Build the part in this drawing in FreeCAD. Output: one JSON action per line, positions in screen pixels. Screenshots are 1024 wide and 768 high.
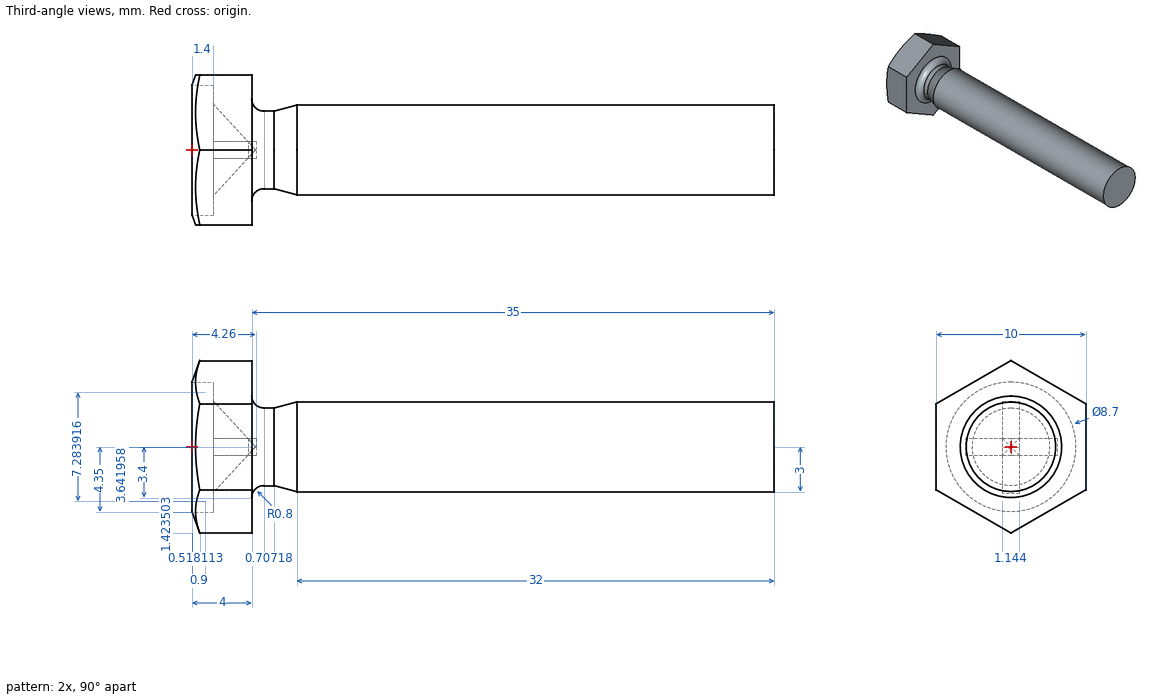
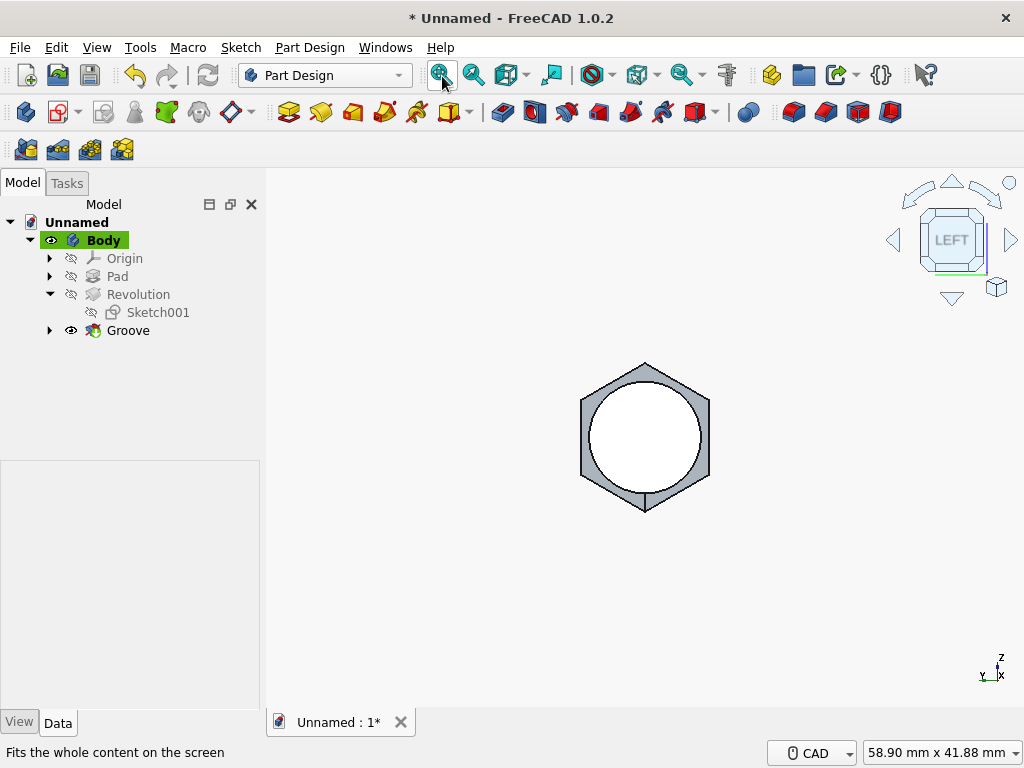
{"action": "key", "text": "v f"}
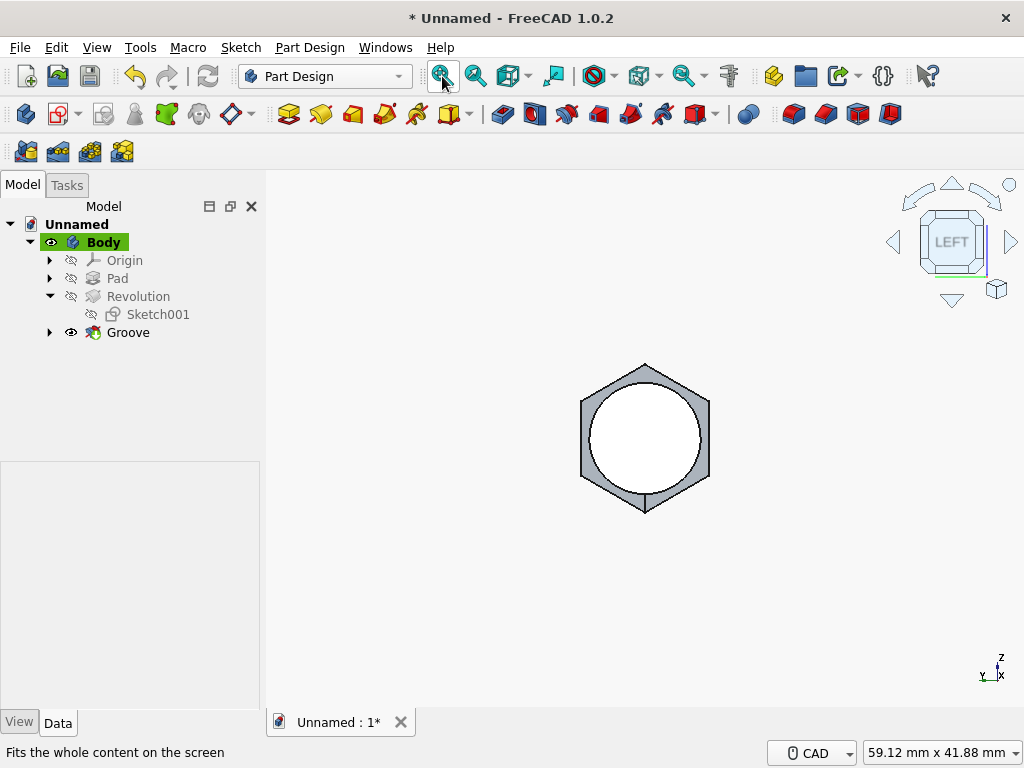
{"action": "left_click", "coordinate": [645, 437]}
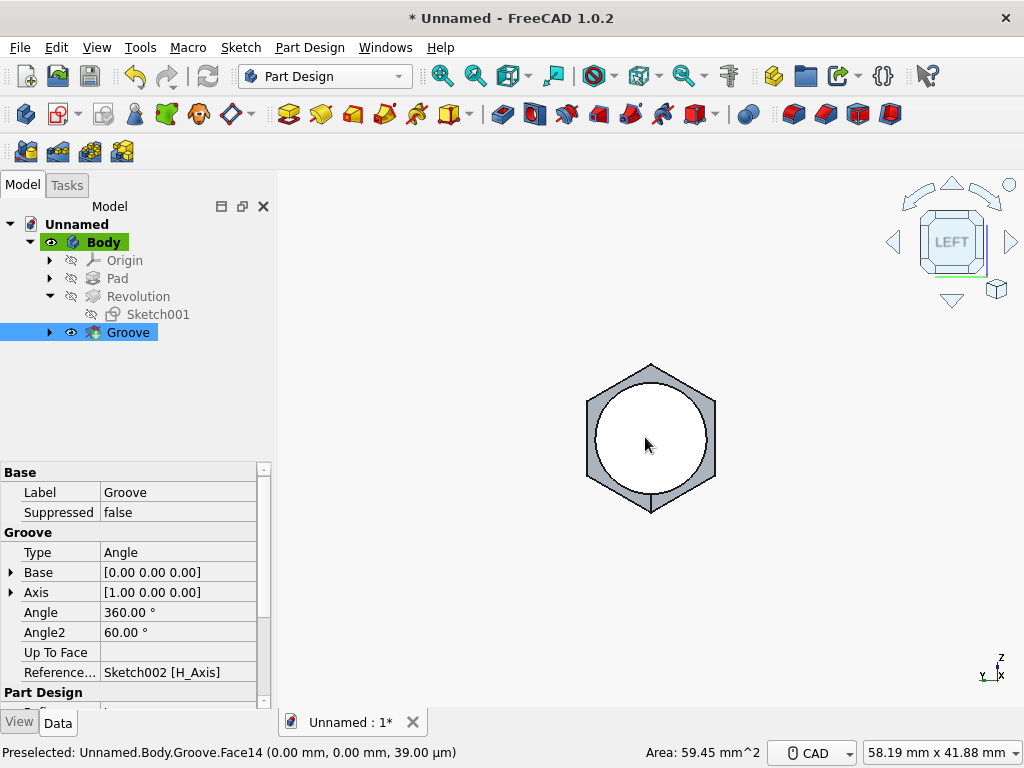
{"action": "left_click", "coordinate": [58, 114]}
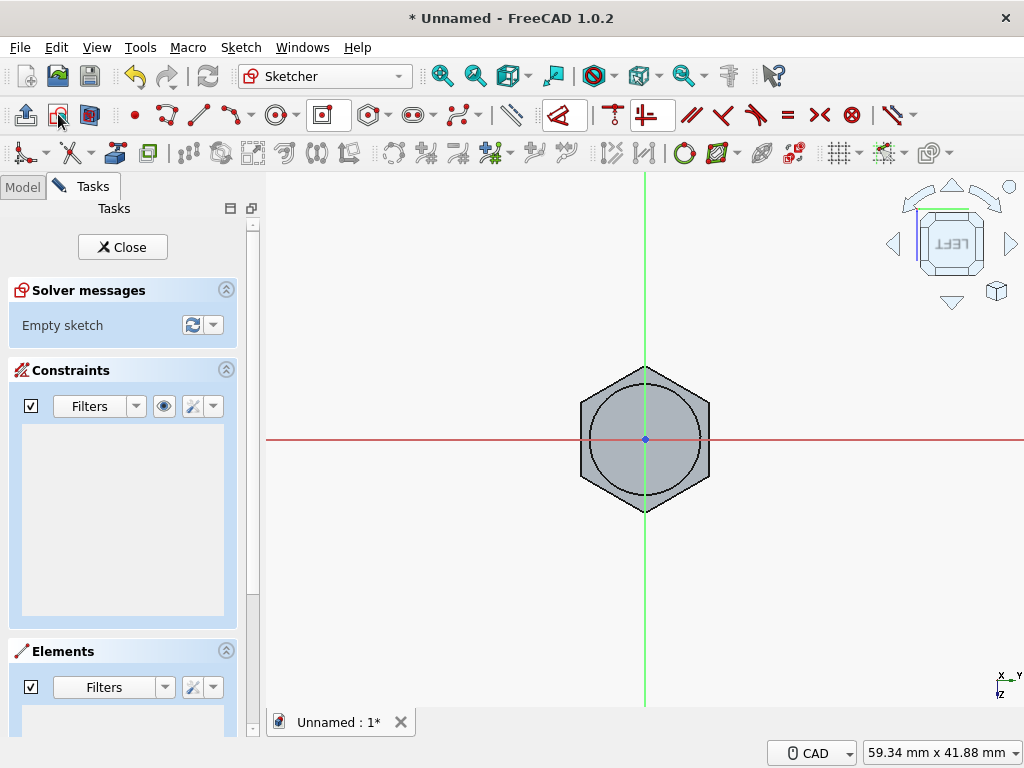
{"action": "scroll", "coordinate": [675, 440], "scroll_direction": "up", "scroll_amount": 6}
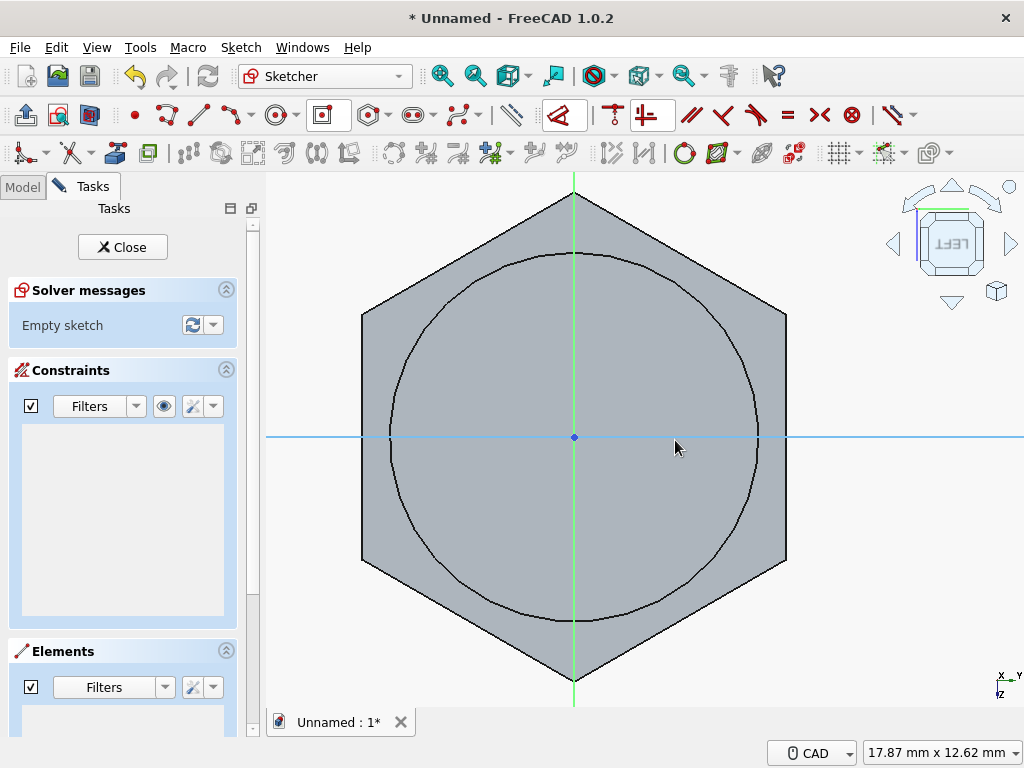
{"action": "left_click", "coordinate": [276, 116]}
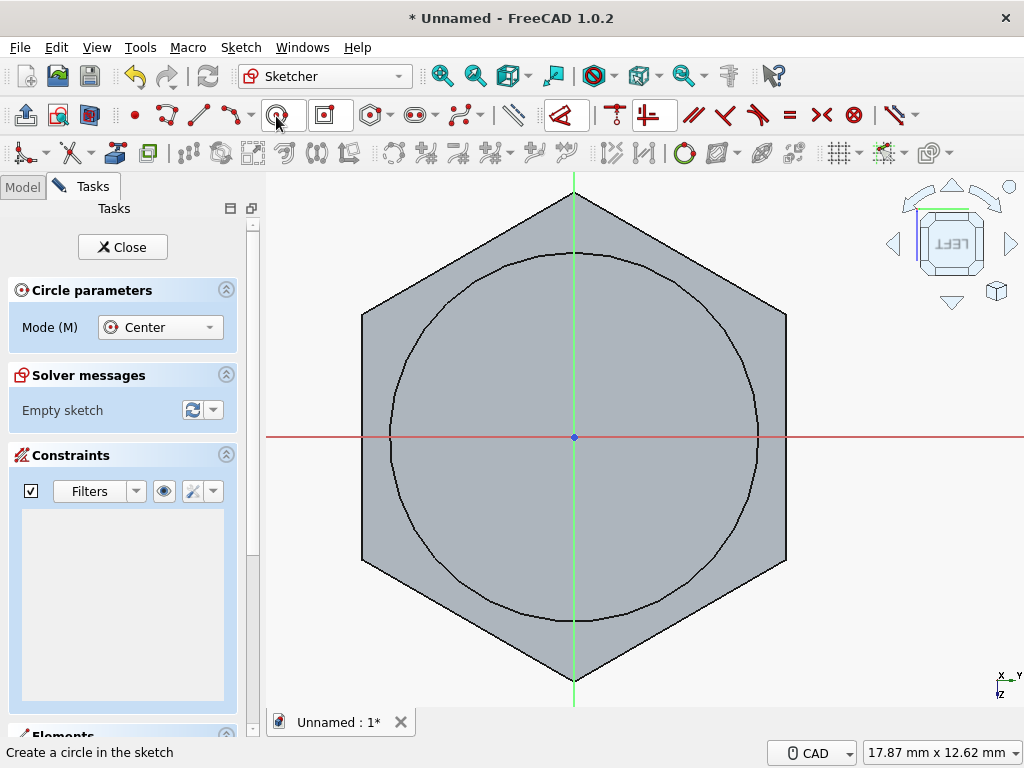
{"action": "left_click", "coordinate": [574, 437]}
{"action": "left_click", "coordinate": [705, 307]}
{"action": "key", "text": "Escape"}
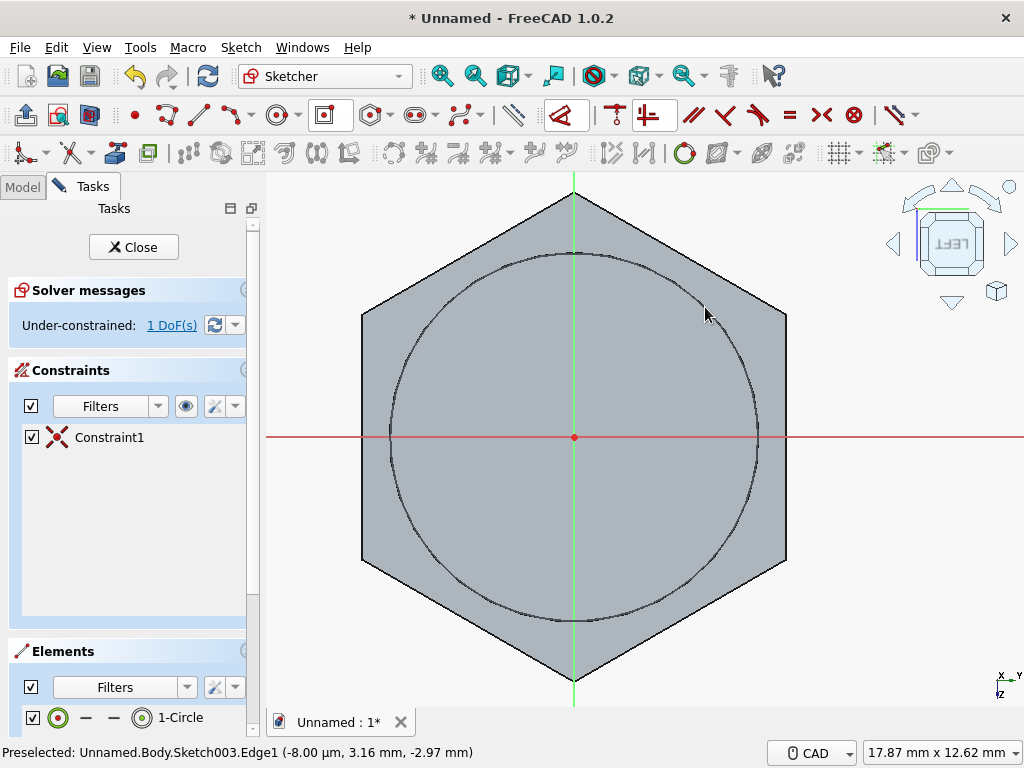
{"action": "left_click", "coordinate": [704, 307]}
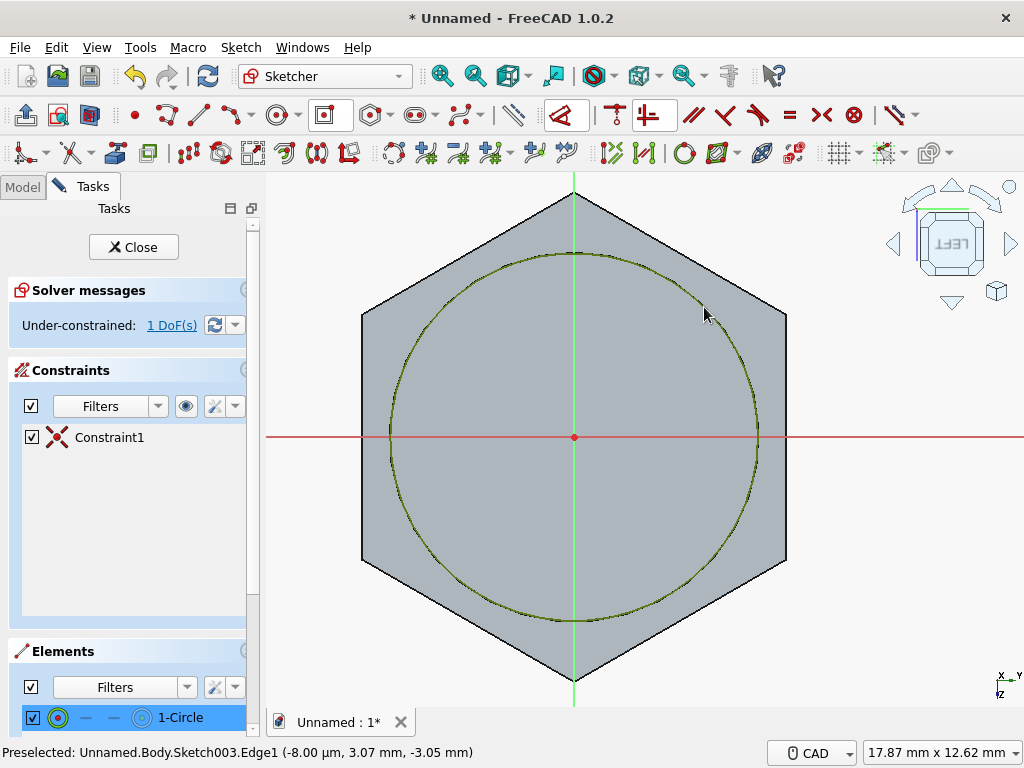
{"action": "left_click", "coordinate": [584, 116]}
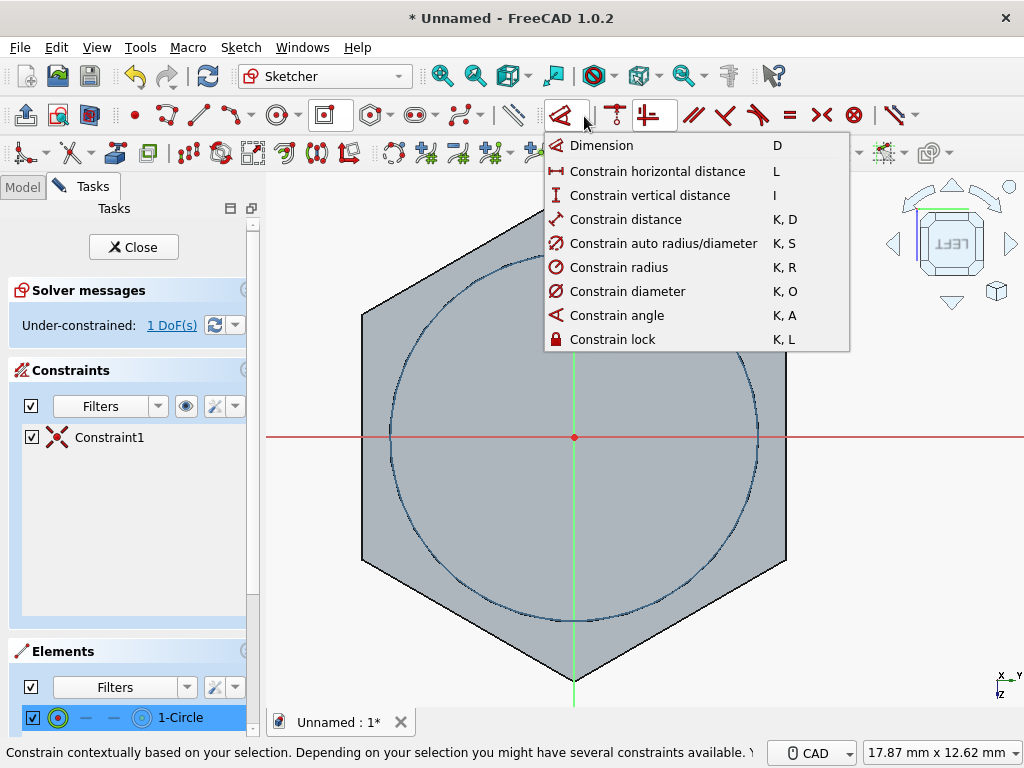
{"action": "left_click", "coordinate": [697, 291]}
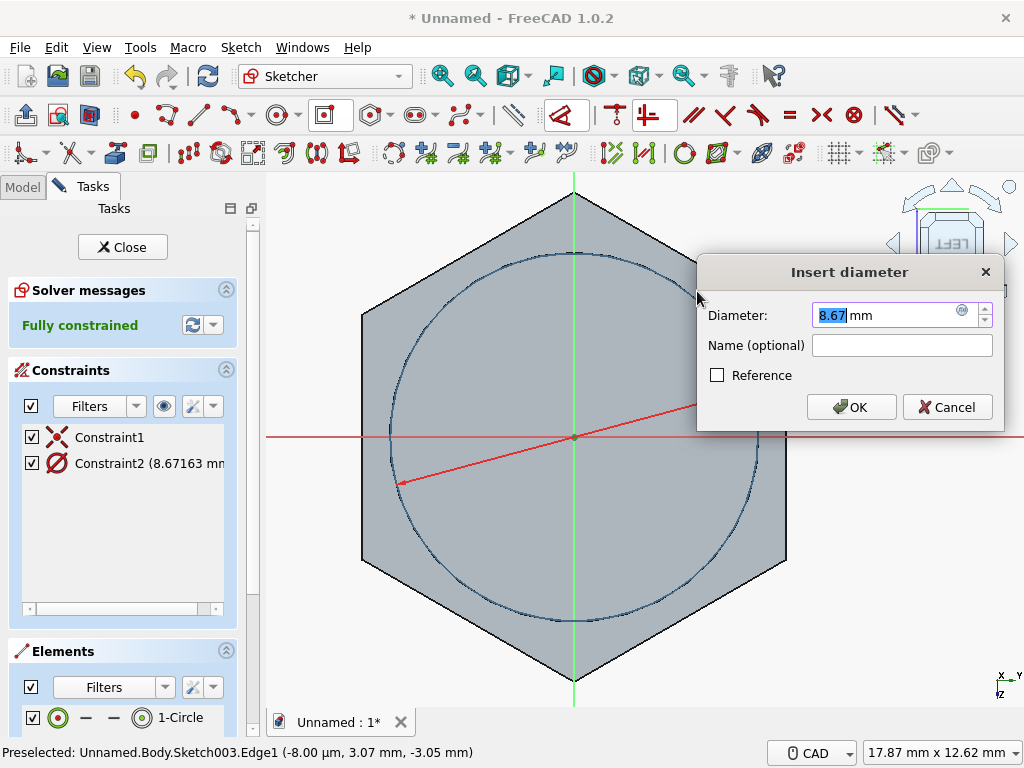
{"action": "type", "text": "8.7"}
{"action": "key", "text": "Return"}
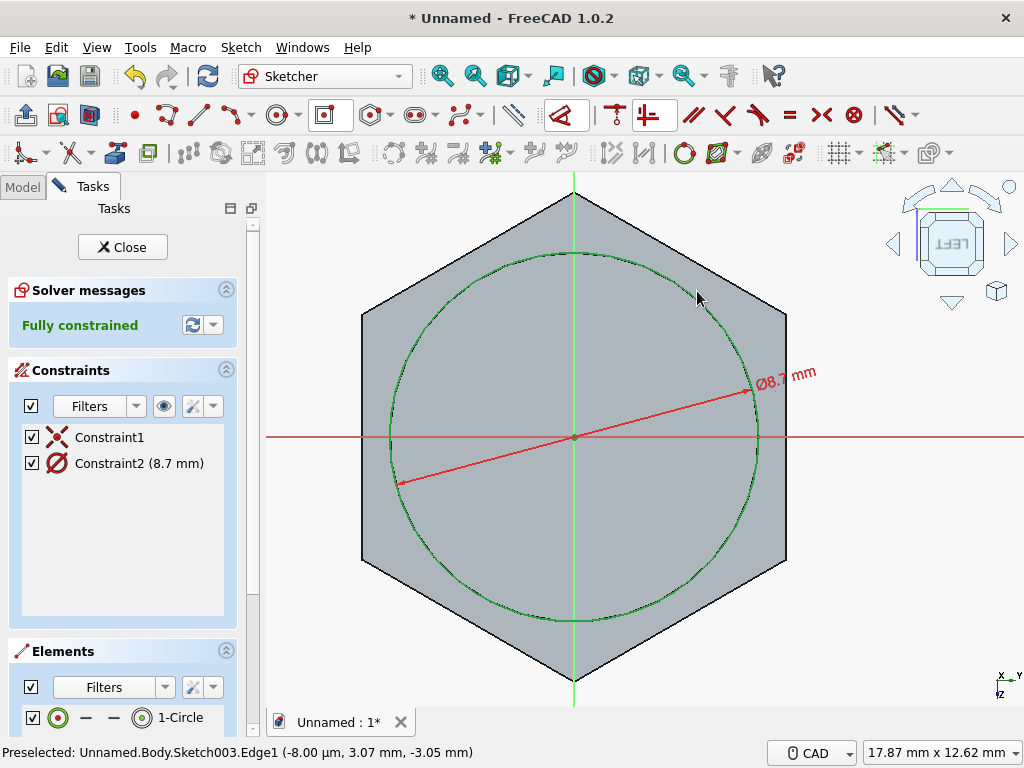
{"action": "left_click", "coordinate": [123, 247]}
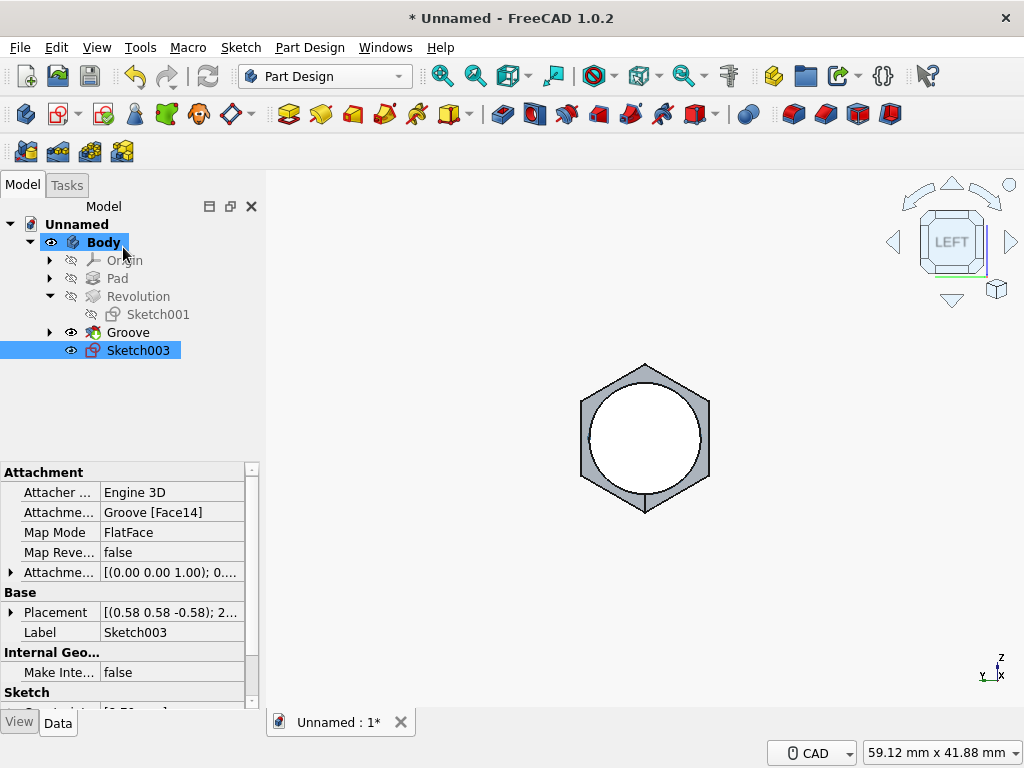
{"action": "left_click", "coordinate": [504, 114]}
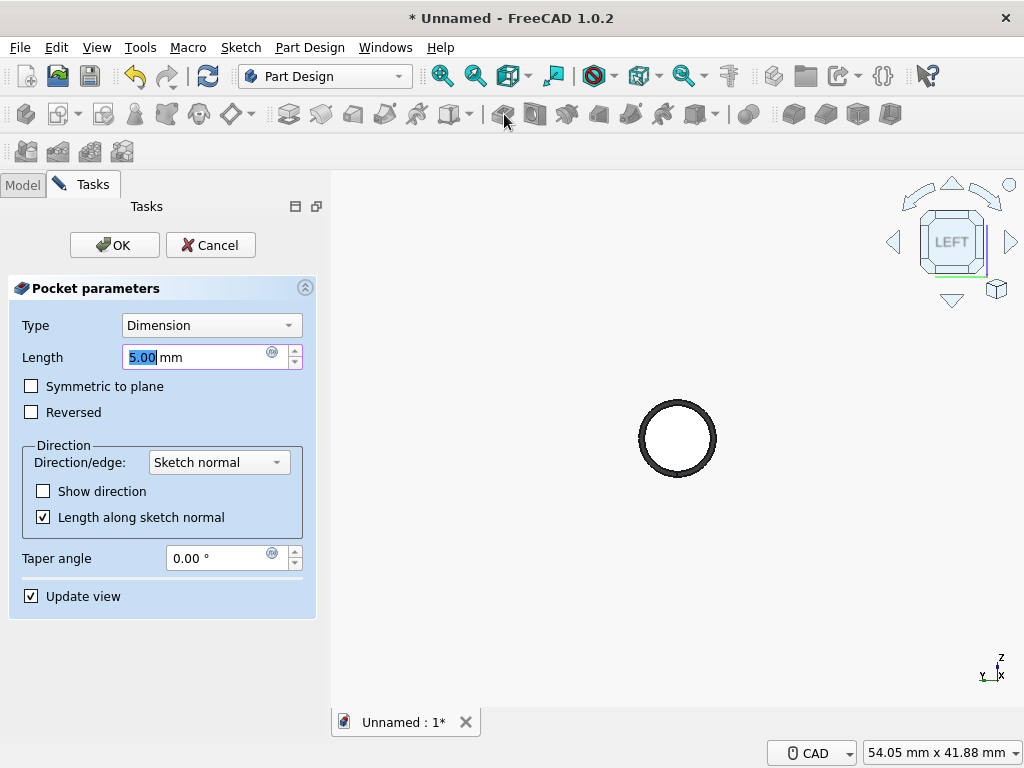
{"action": "type", "text": "1.4"}
{"action": "key", "text": "Tab"}